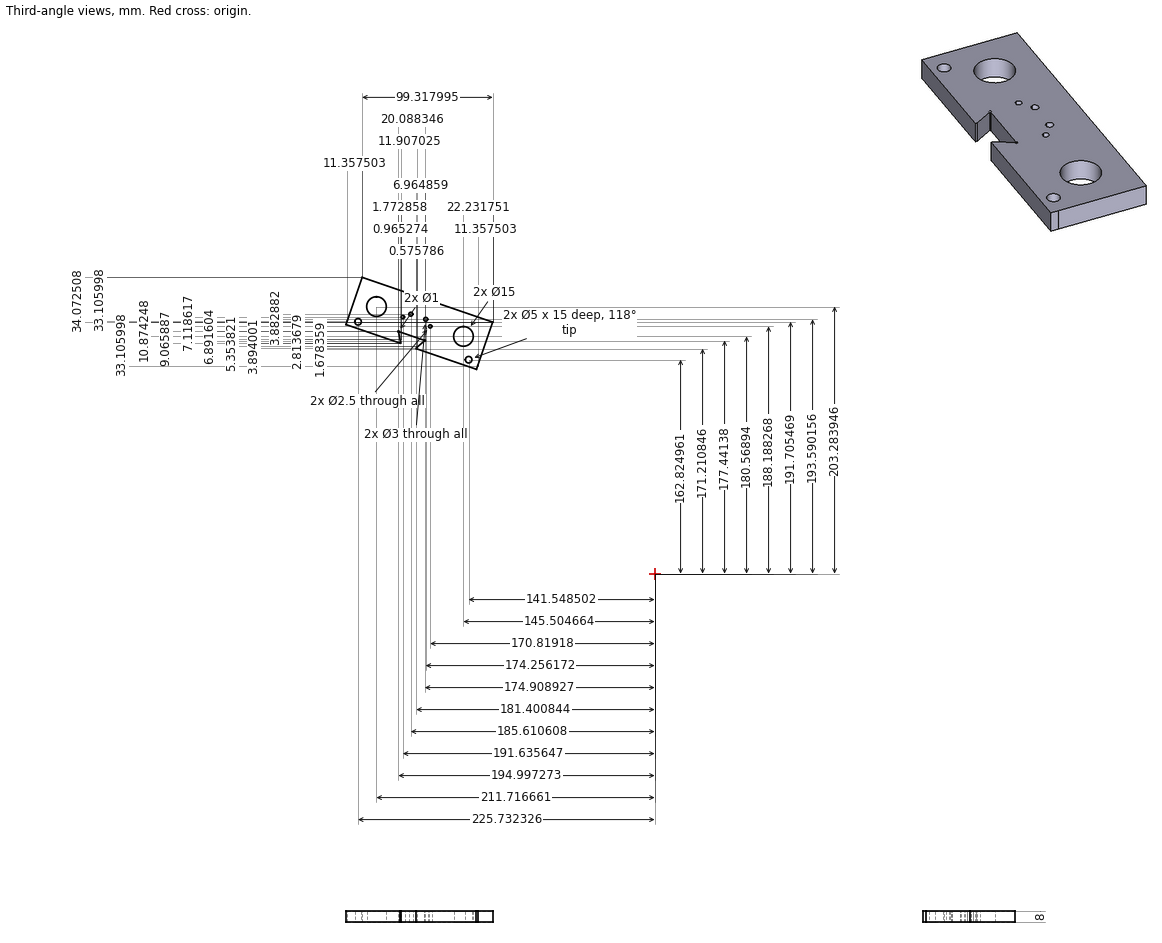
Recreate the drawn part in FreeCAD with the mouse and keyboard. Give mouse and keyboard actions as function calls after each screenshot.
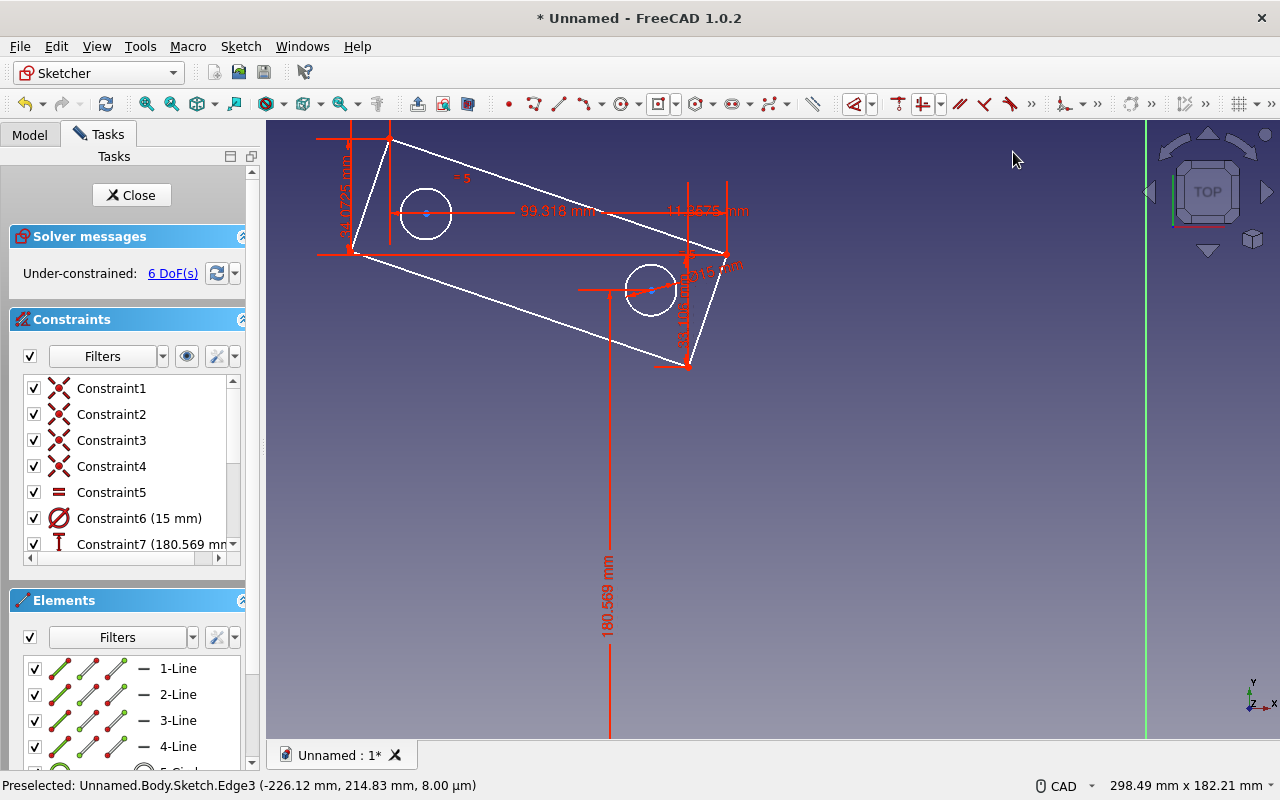
click(378, 173)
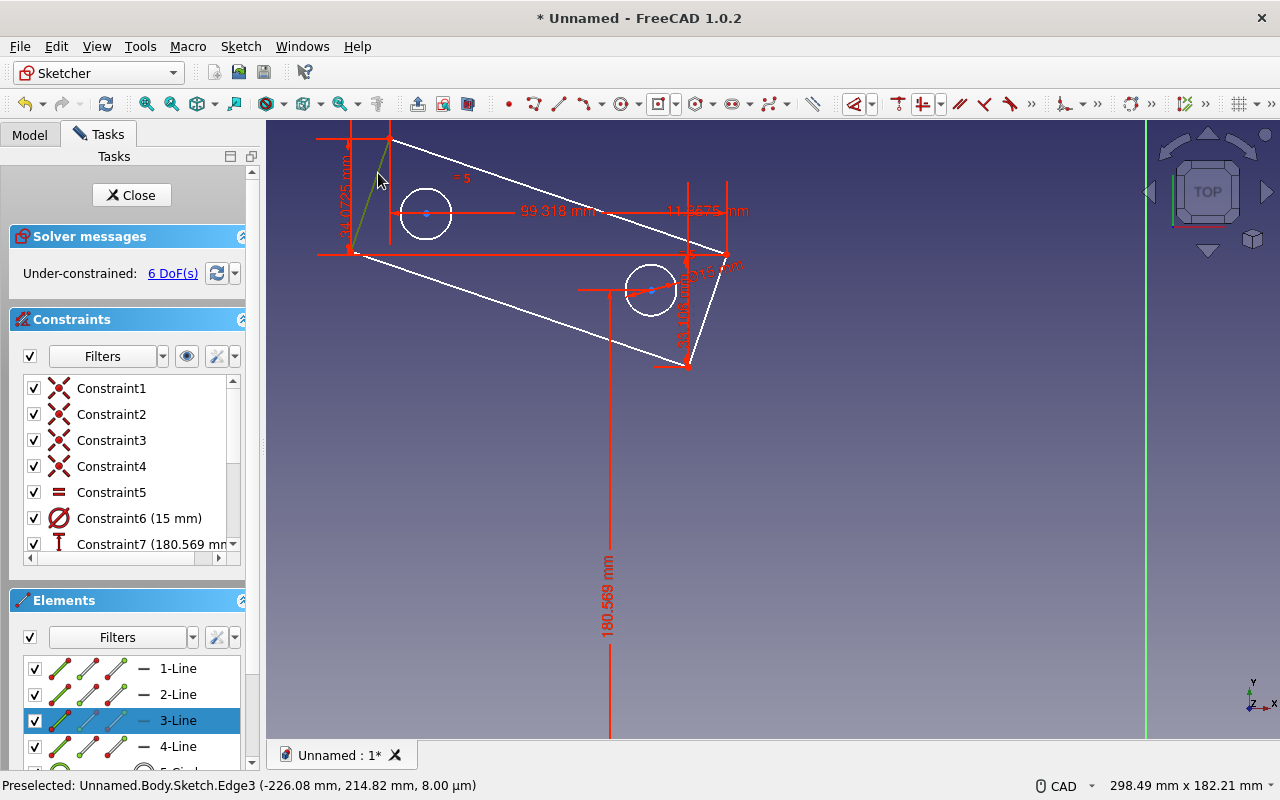
click(872, 104)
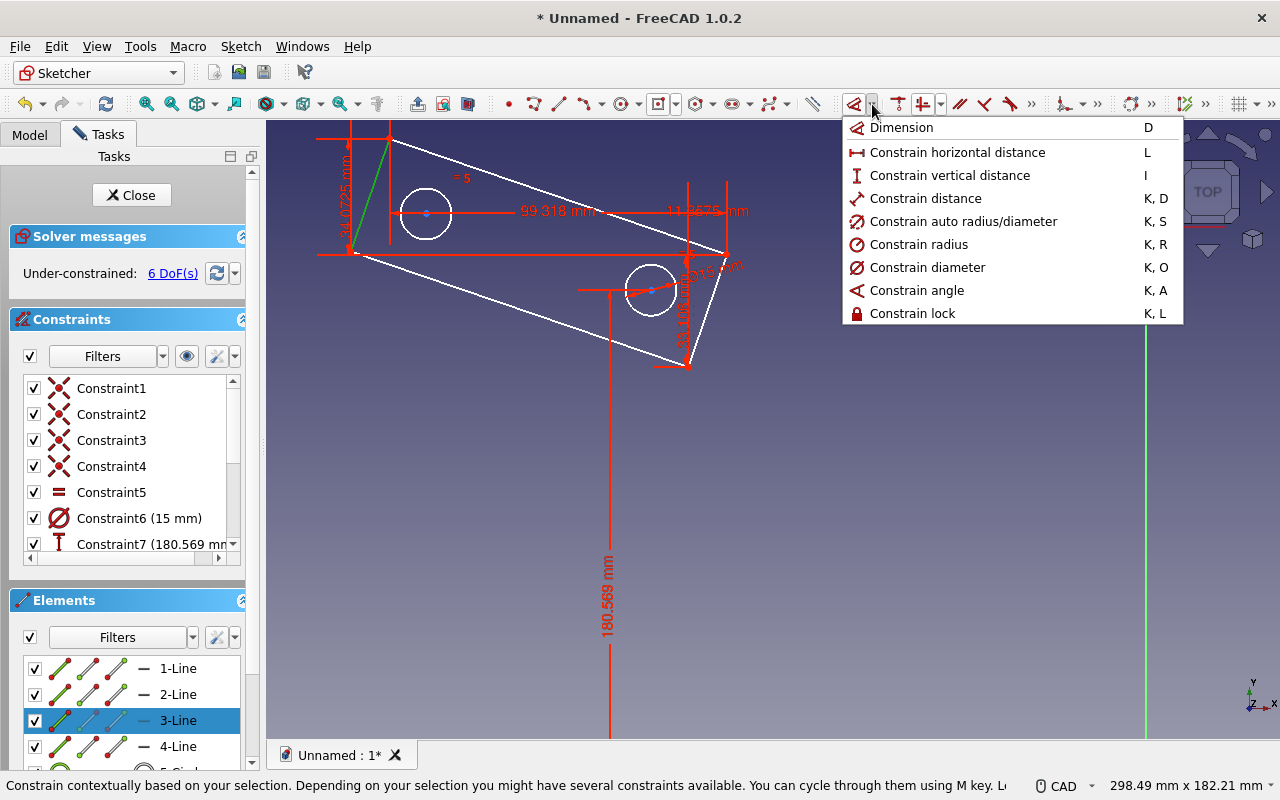
click(1013, 176)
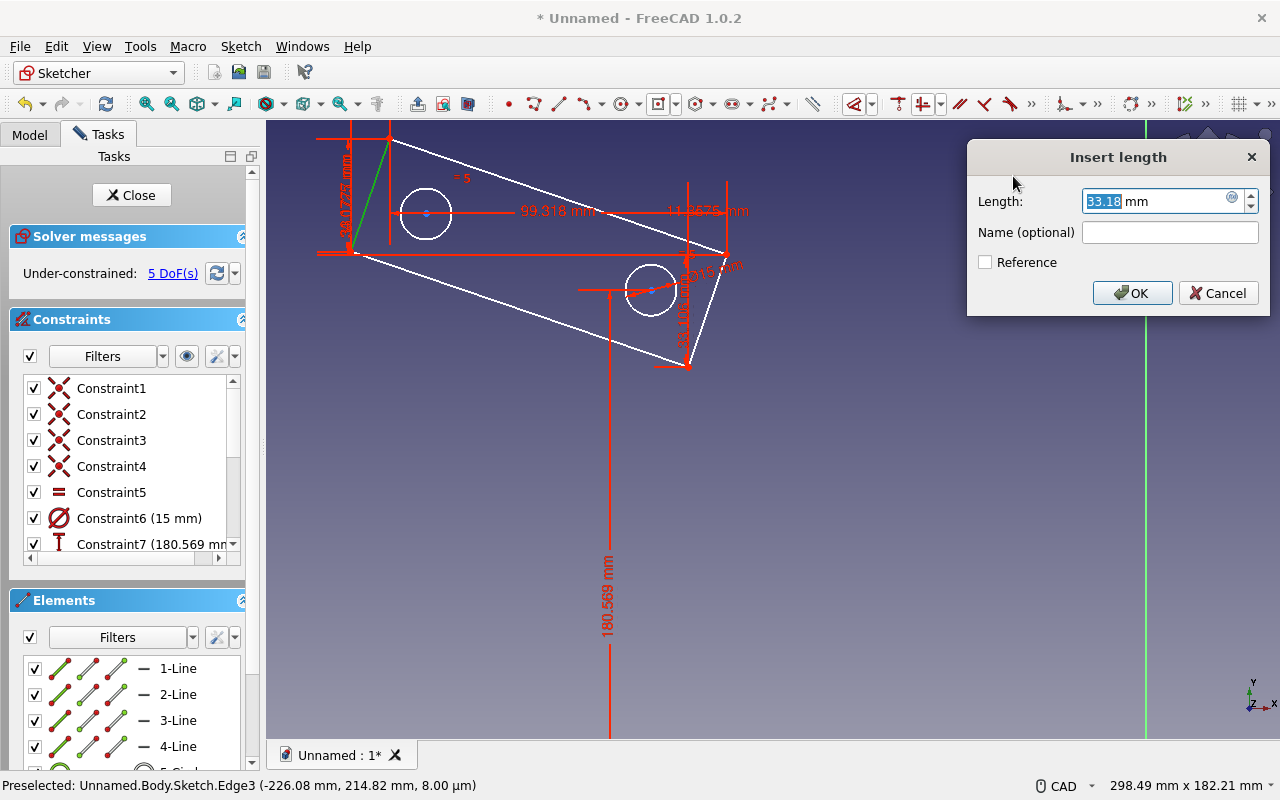
text(33.105998)
key(Return)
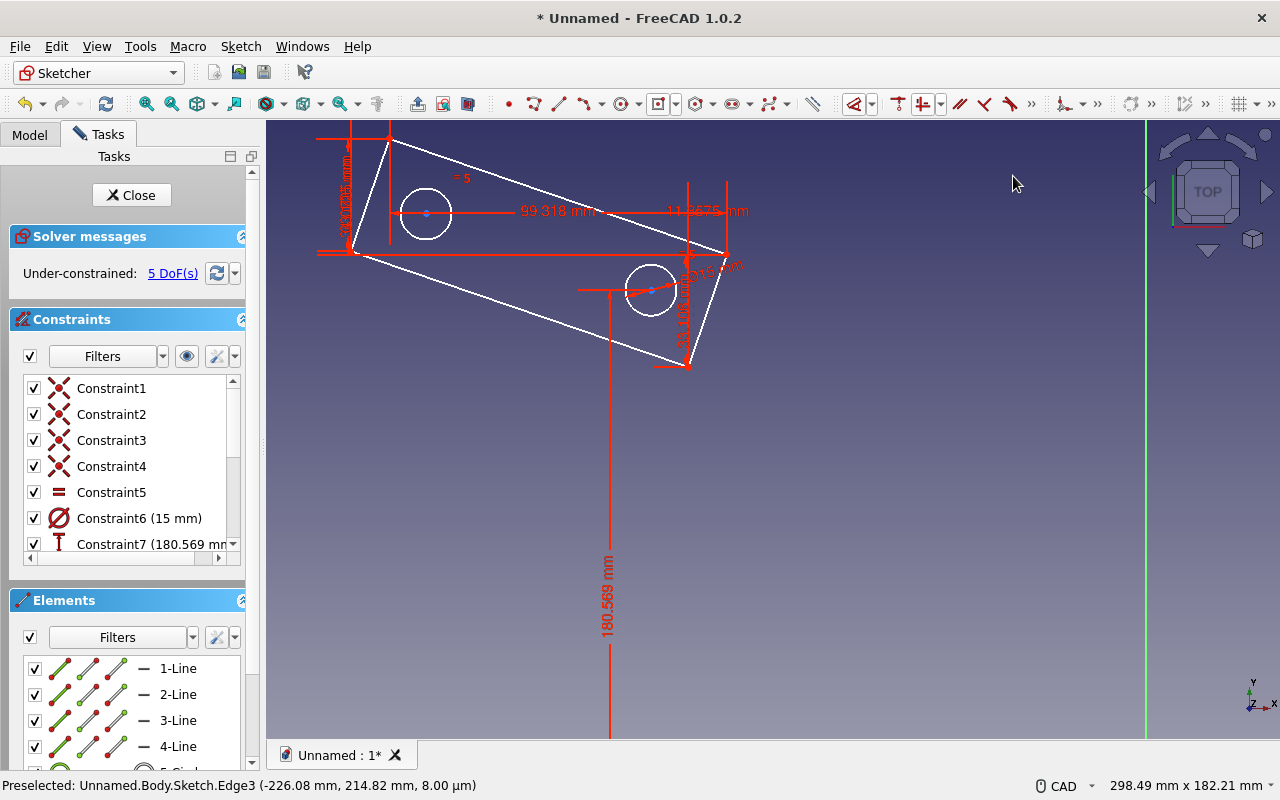
click(651, 290)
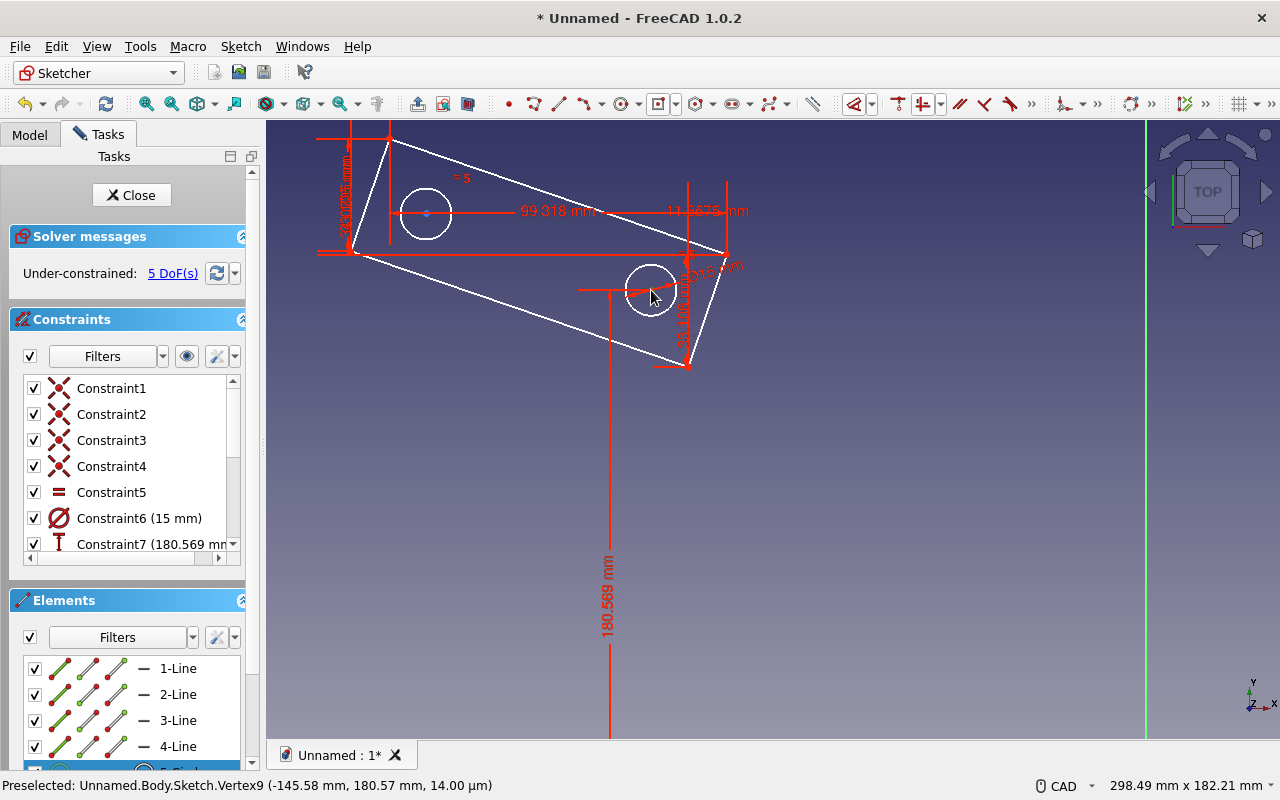
key(l)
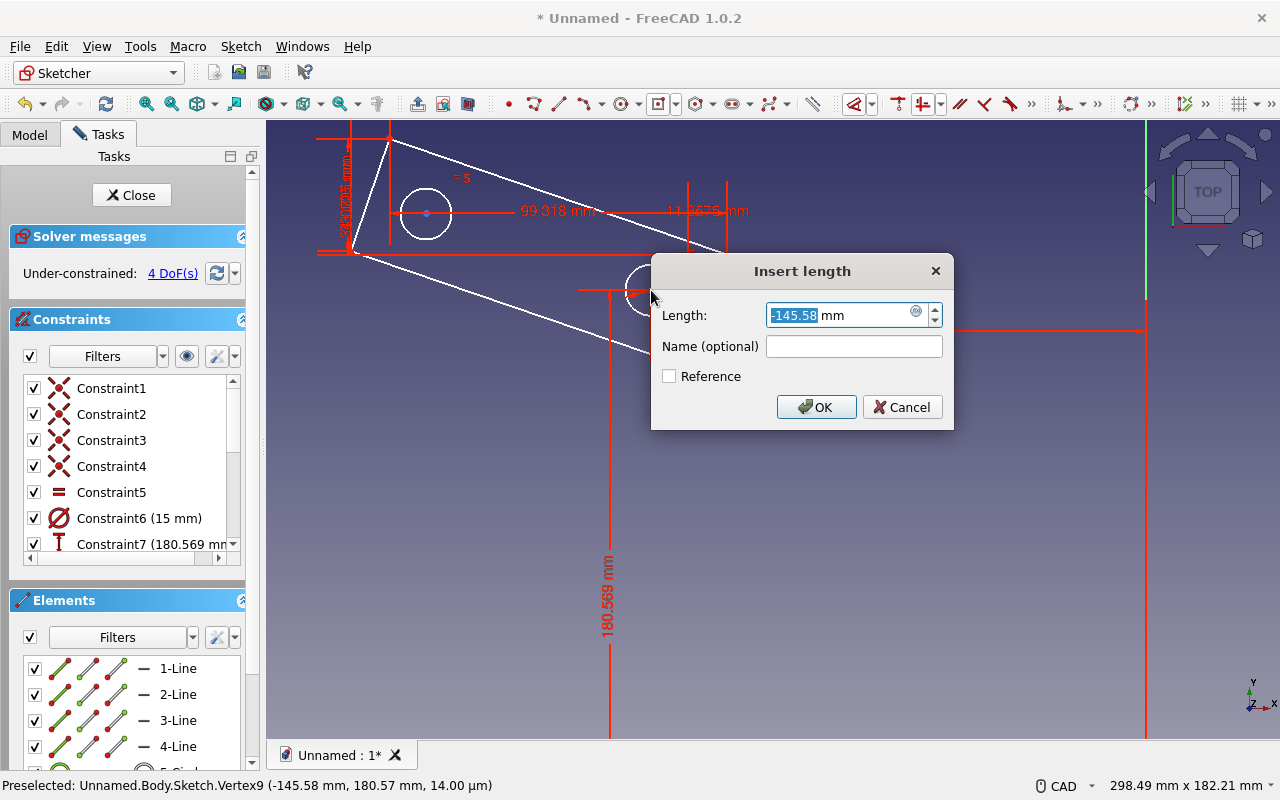
text(-145.504664)
key(Return)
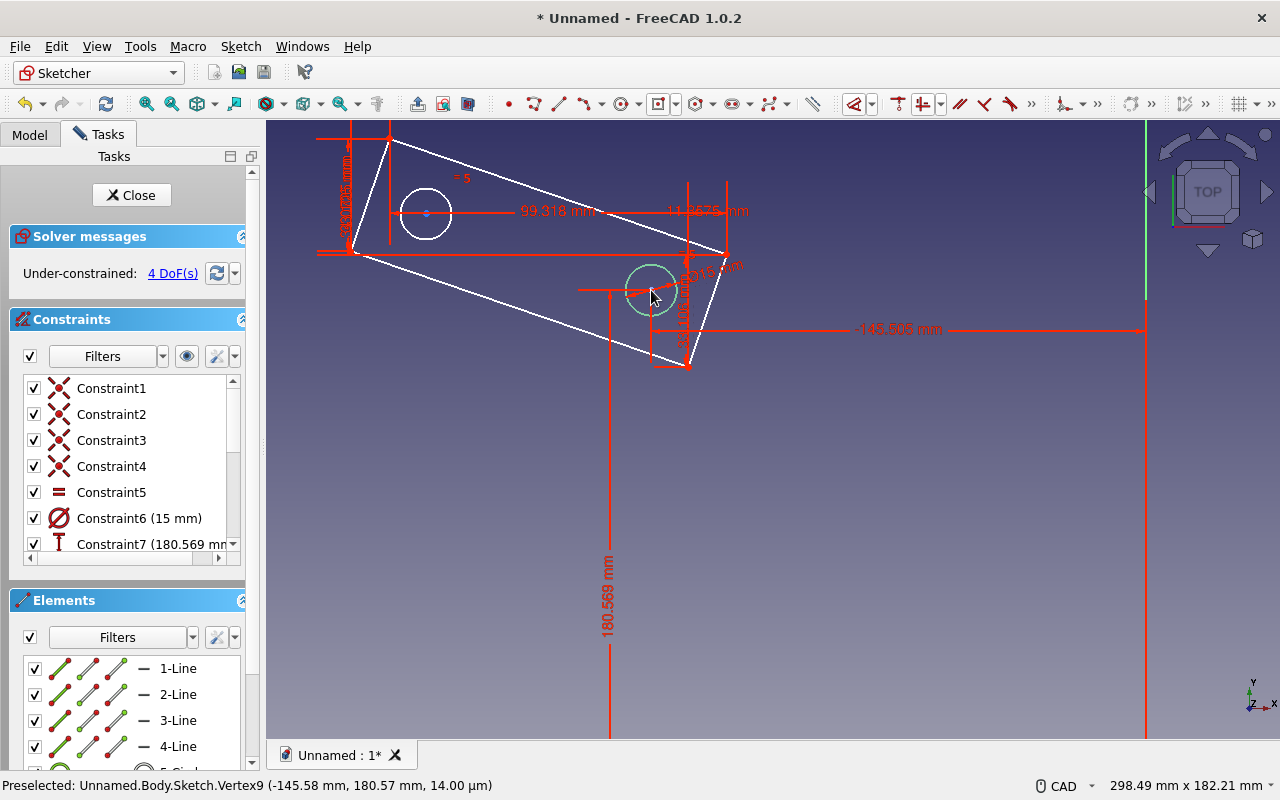
click(426, 214)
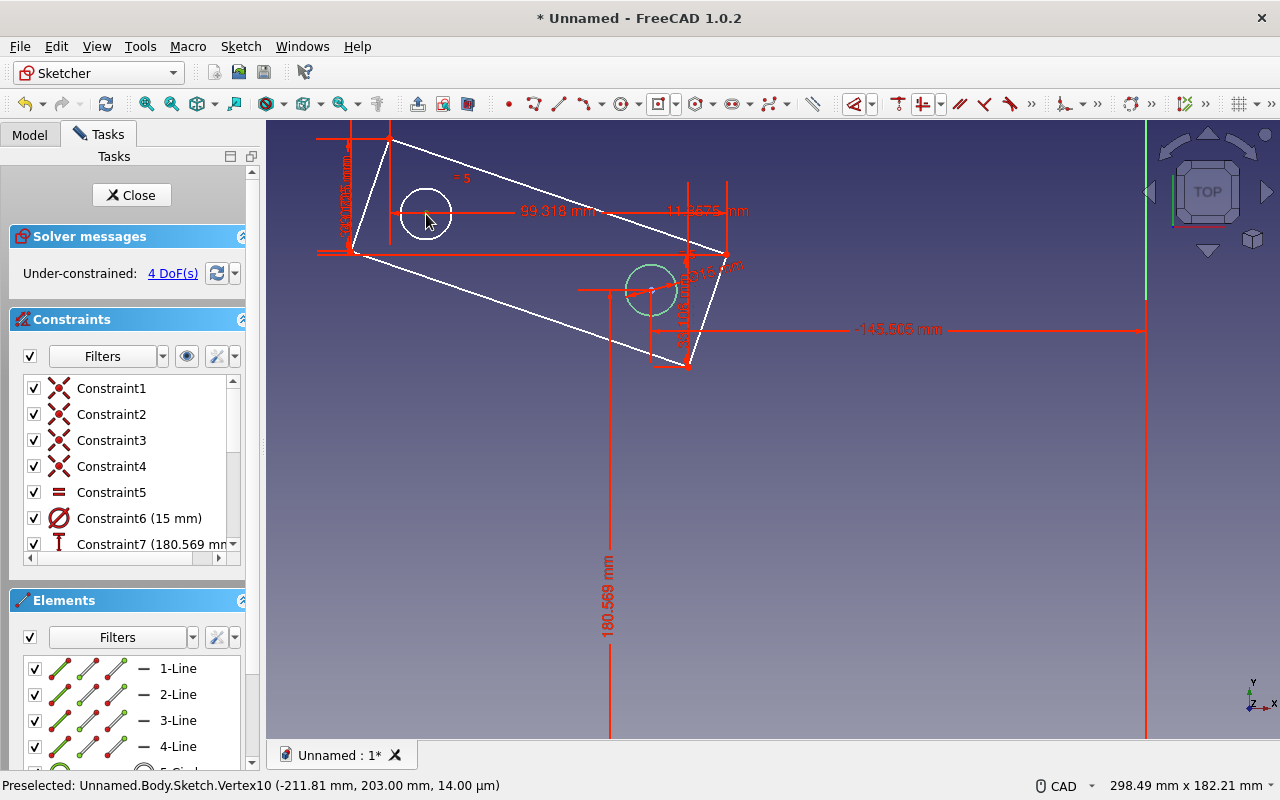
click(872, 104)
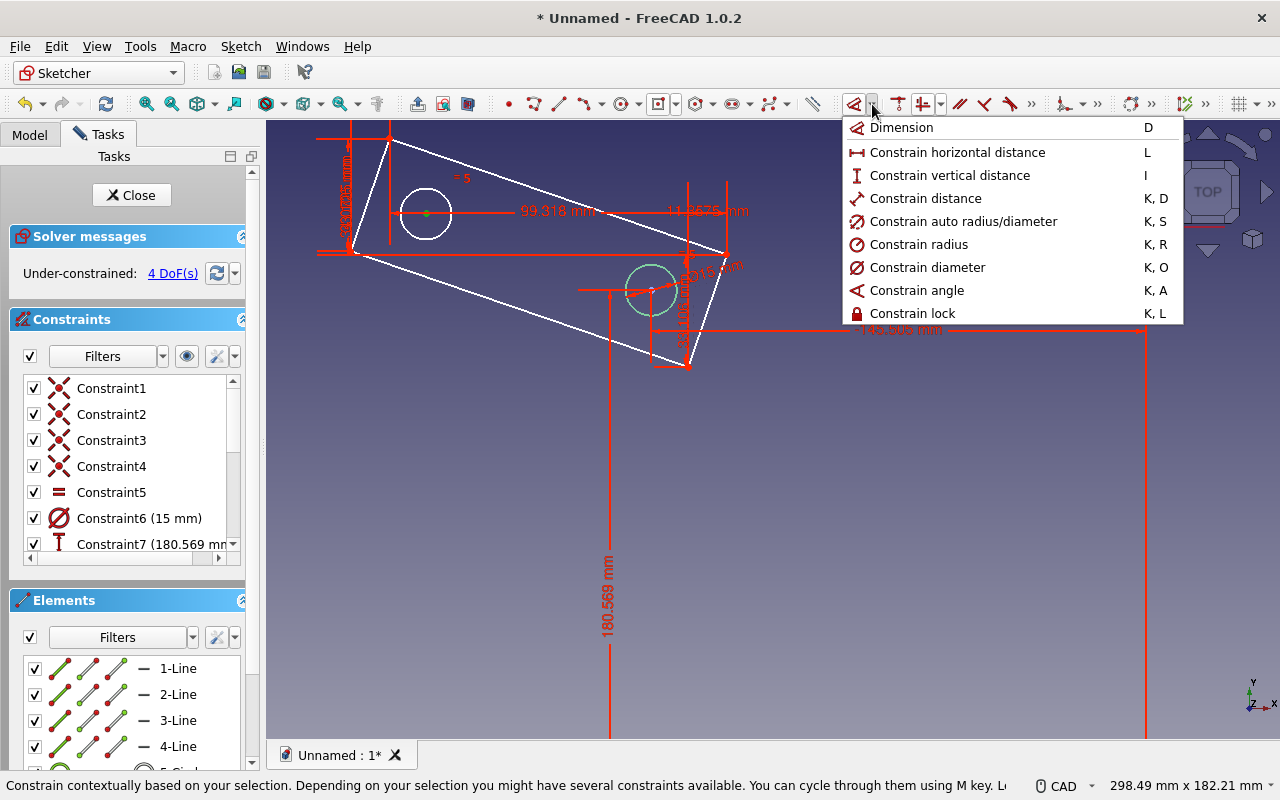
click(1013, 152)